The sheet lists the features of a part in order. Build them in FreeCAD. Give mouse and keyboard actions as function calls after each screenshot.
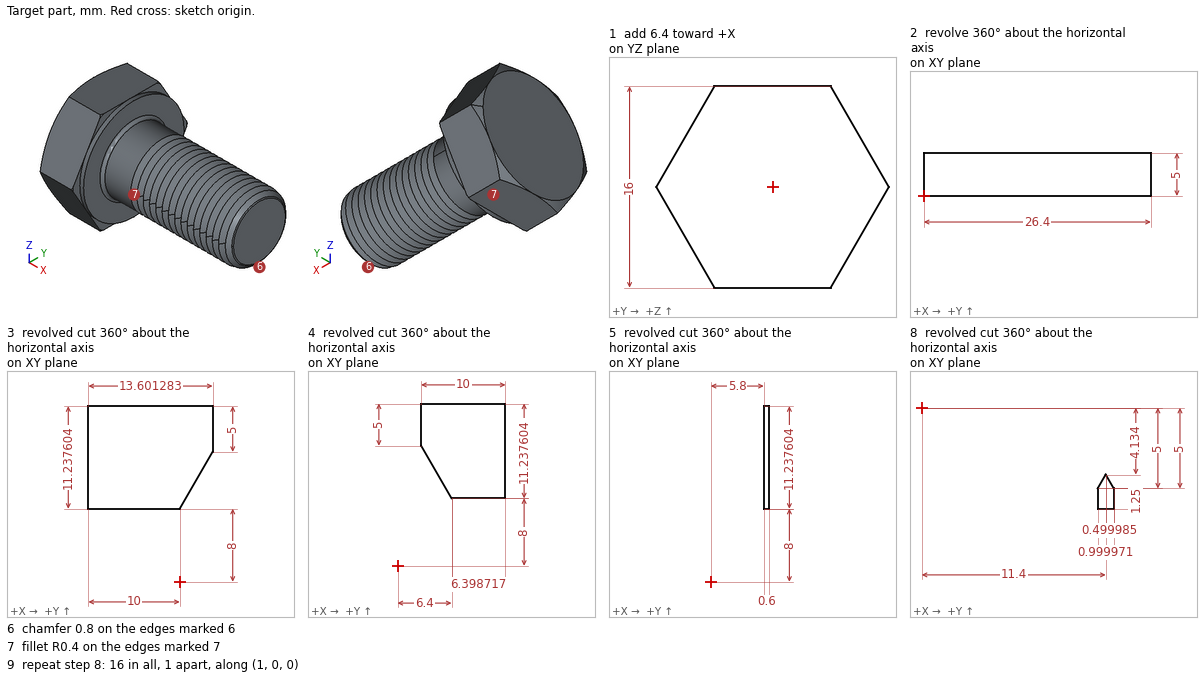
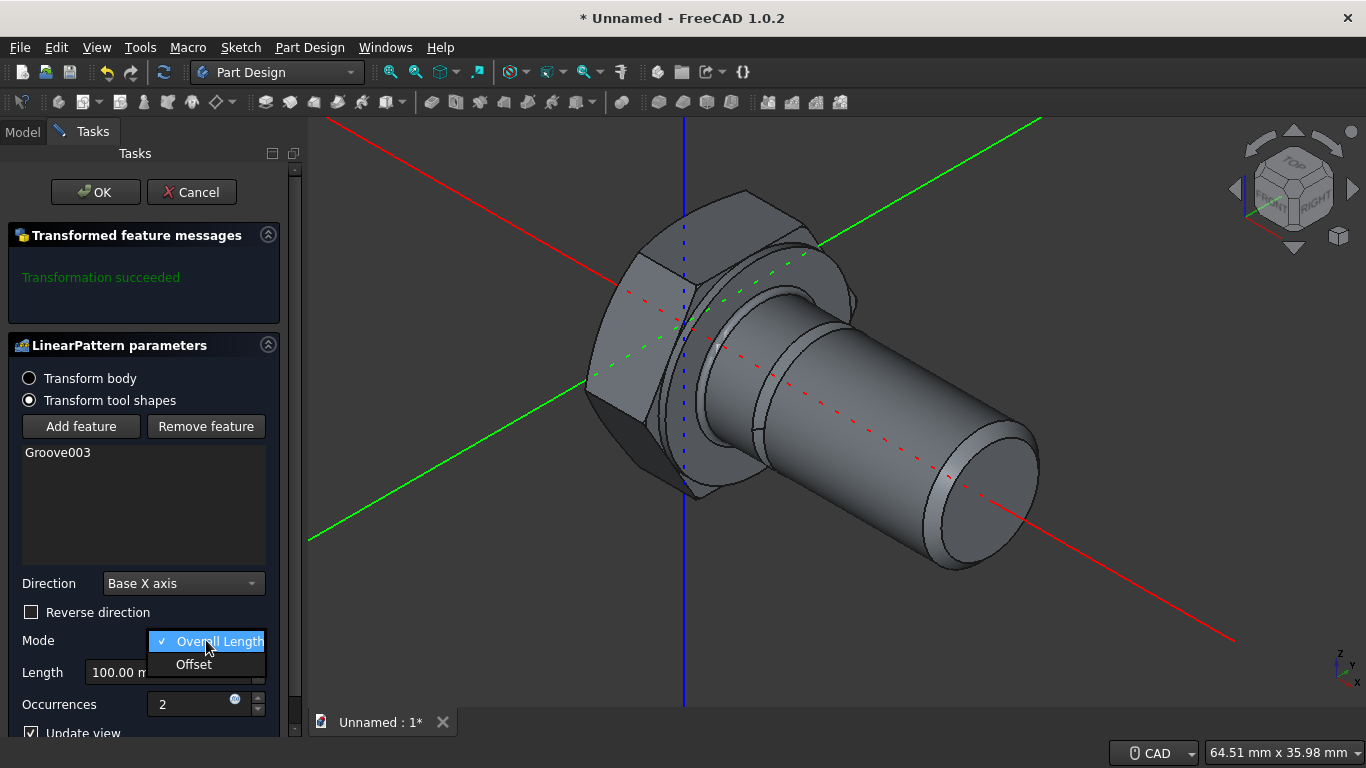
click(206, 664)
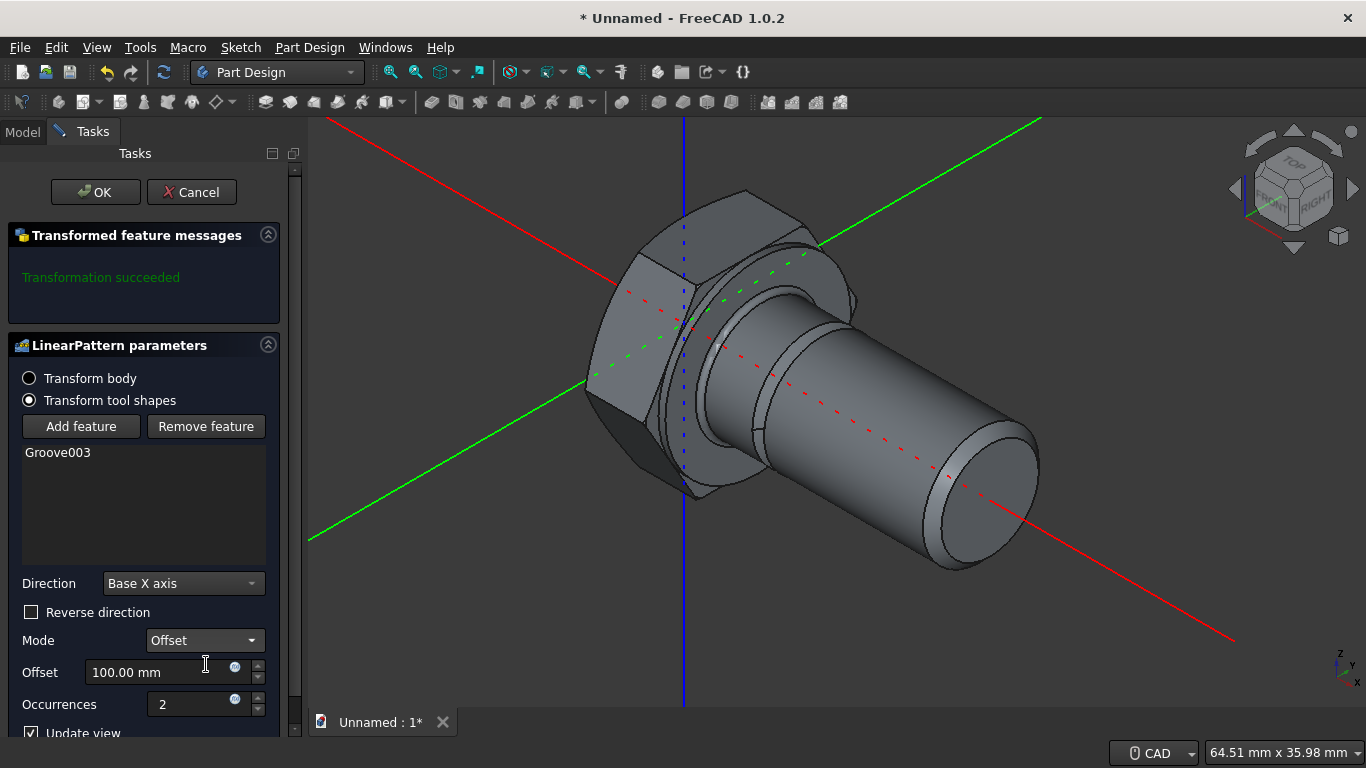
triple_click(168, 672)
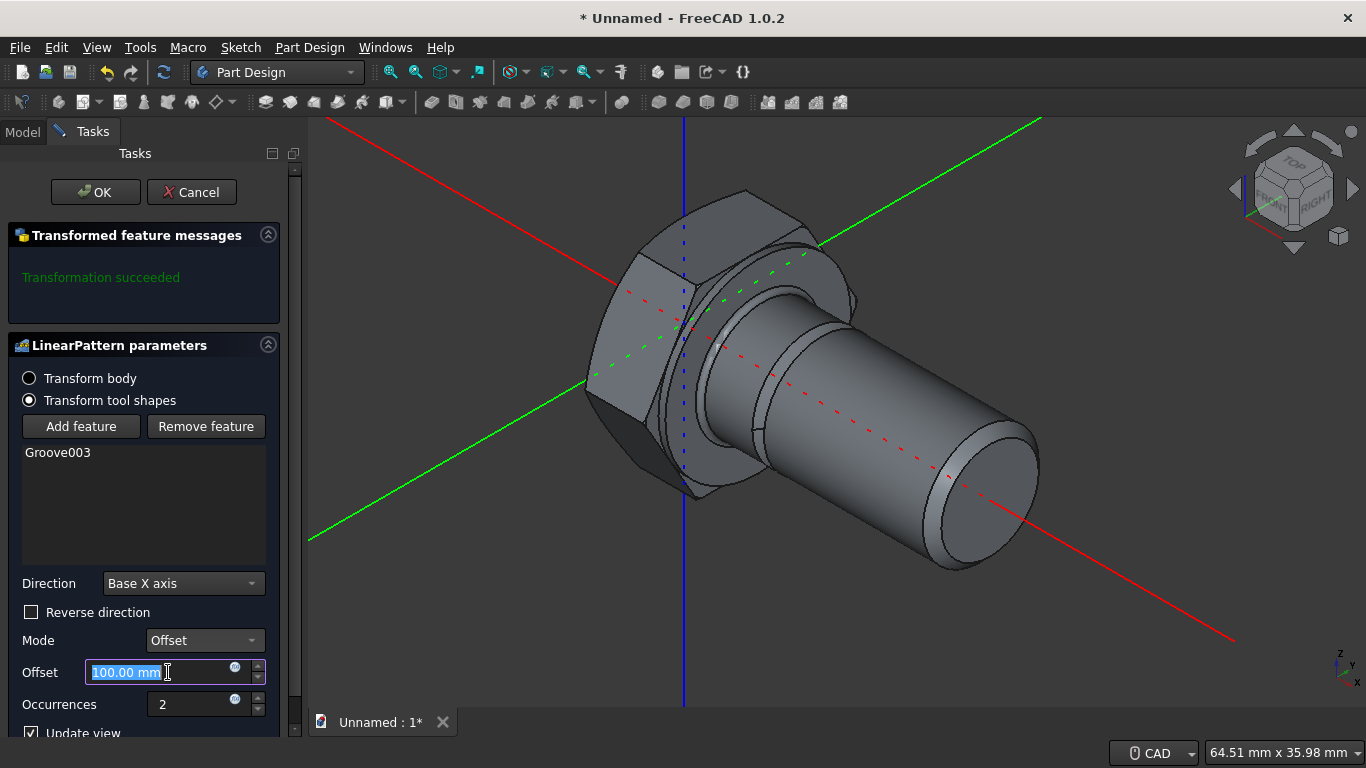
text(1)
key(Tab)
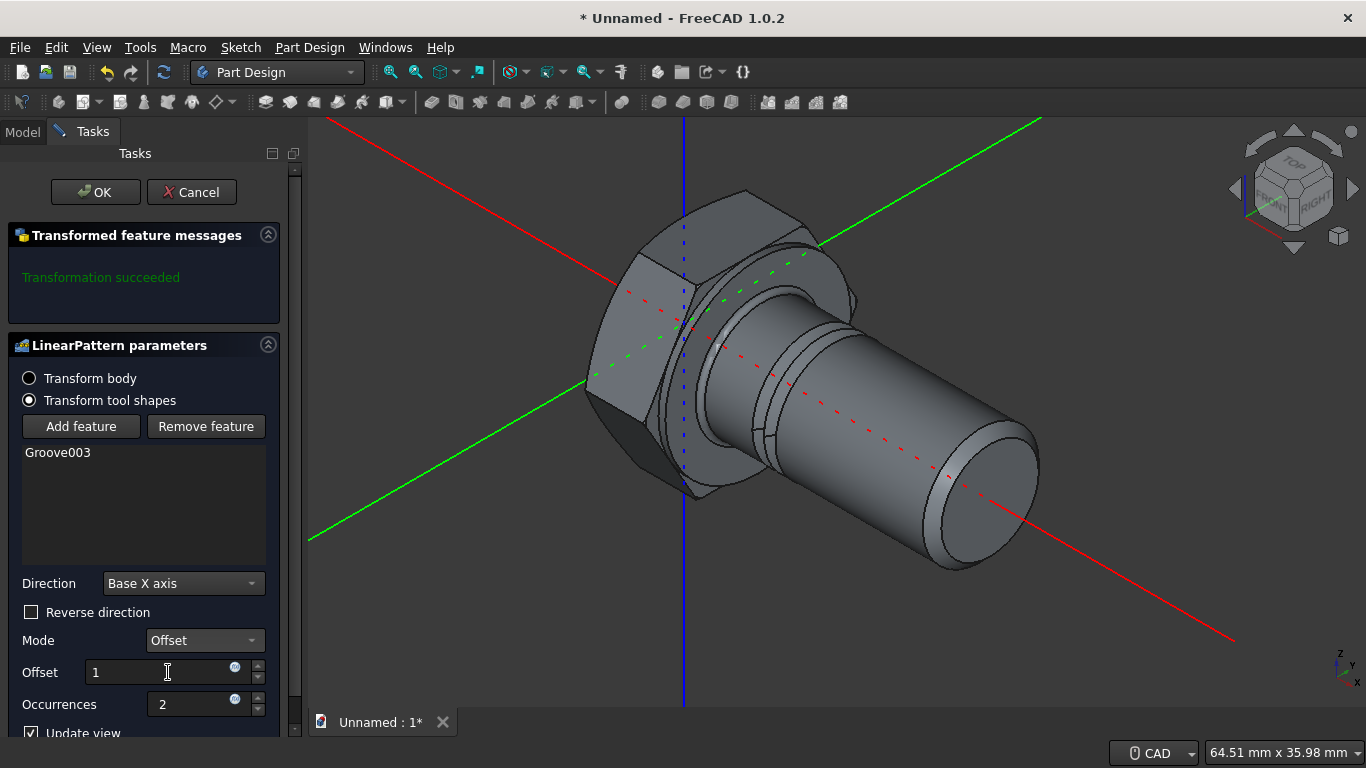
triple_click(198, 704)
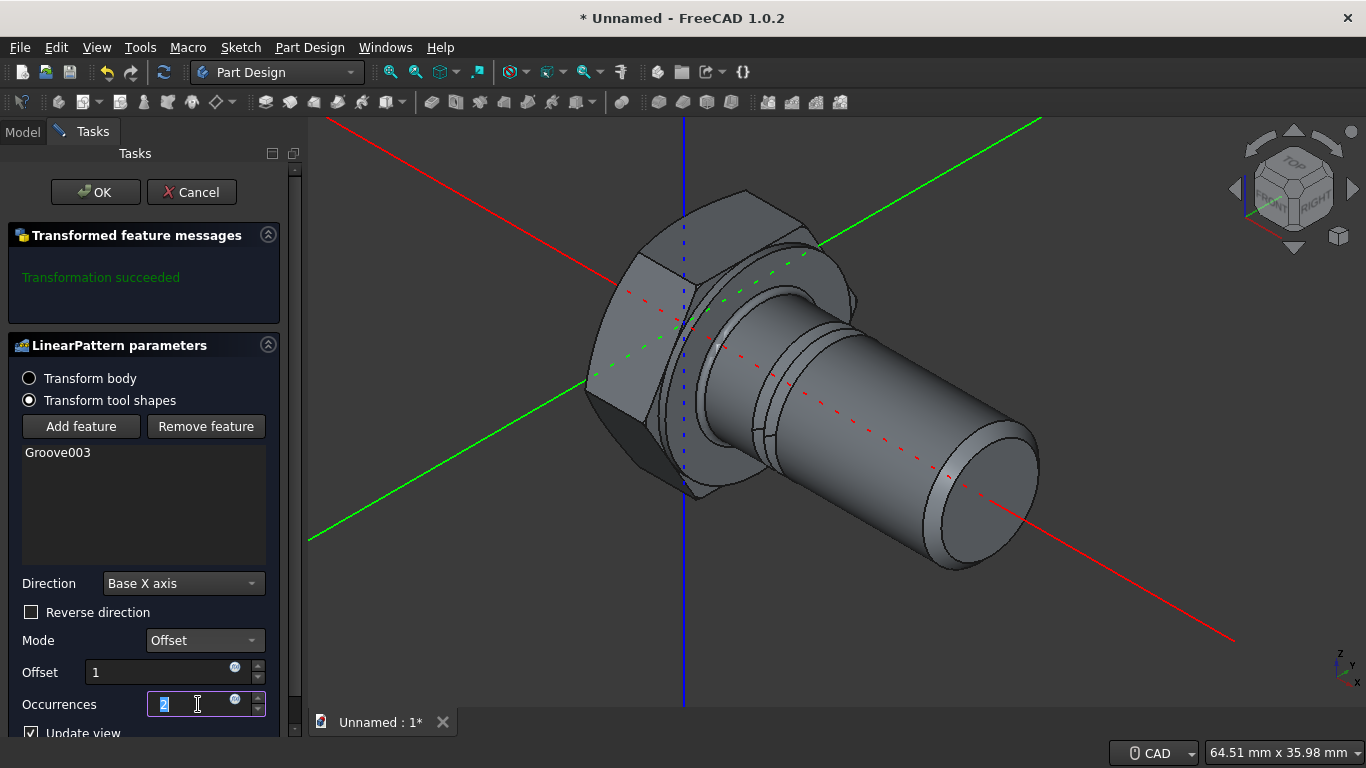
text(16)
key(Tab)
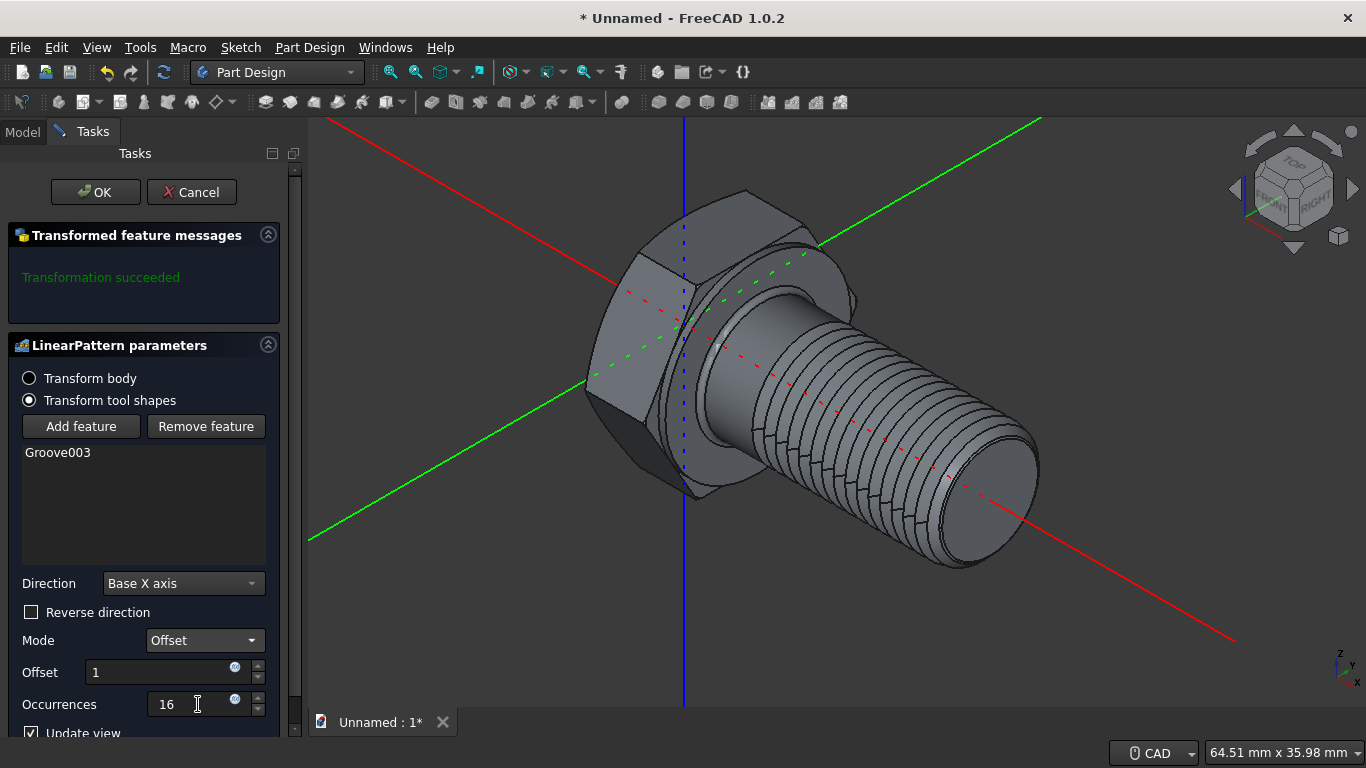
click(96, 192)